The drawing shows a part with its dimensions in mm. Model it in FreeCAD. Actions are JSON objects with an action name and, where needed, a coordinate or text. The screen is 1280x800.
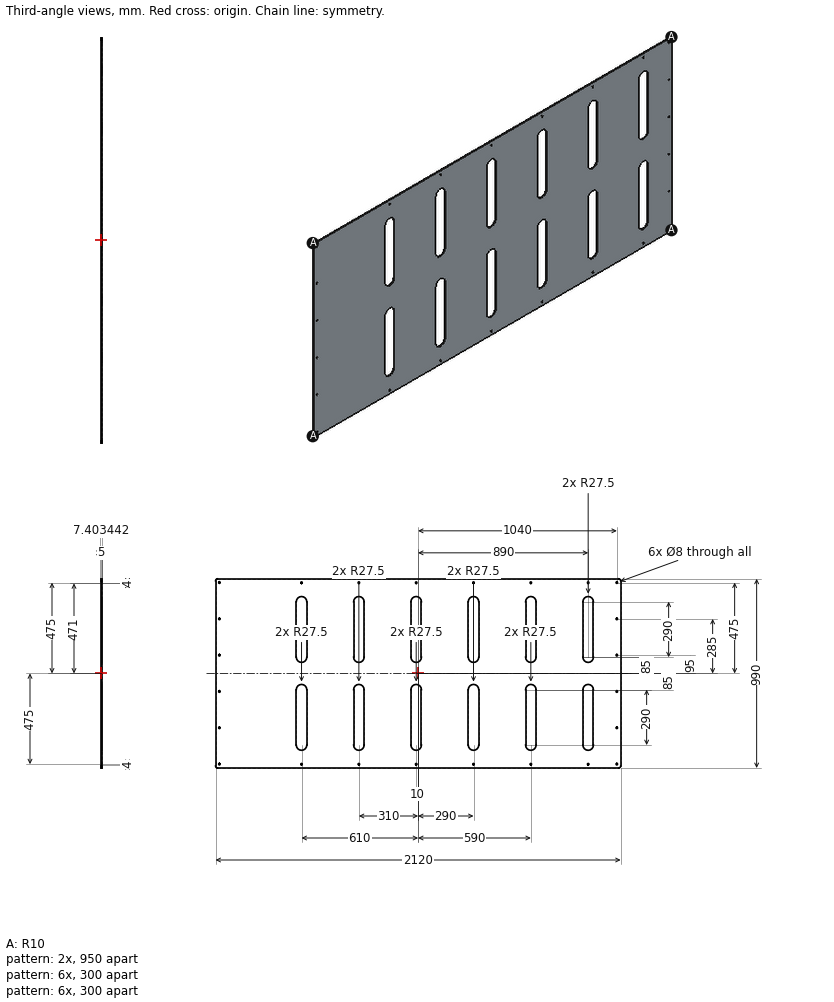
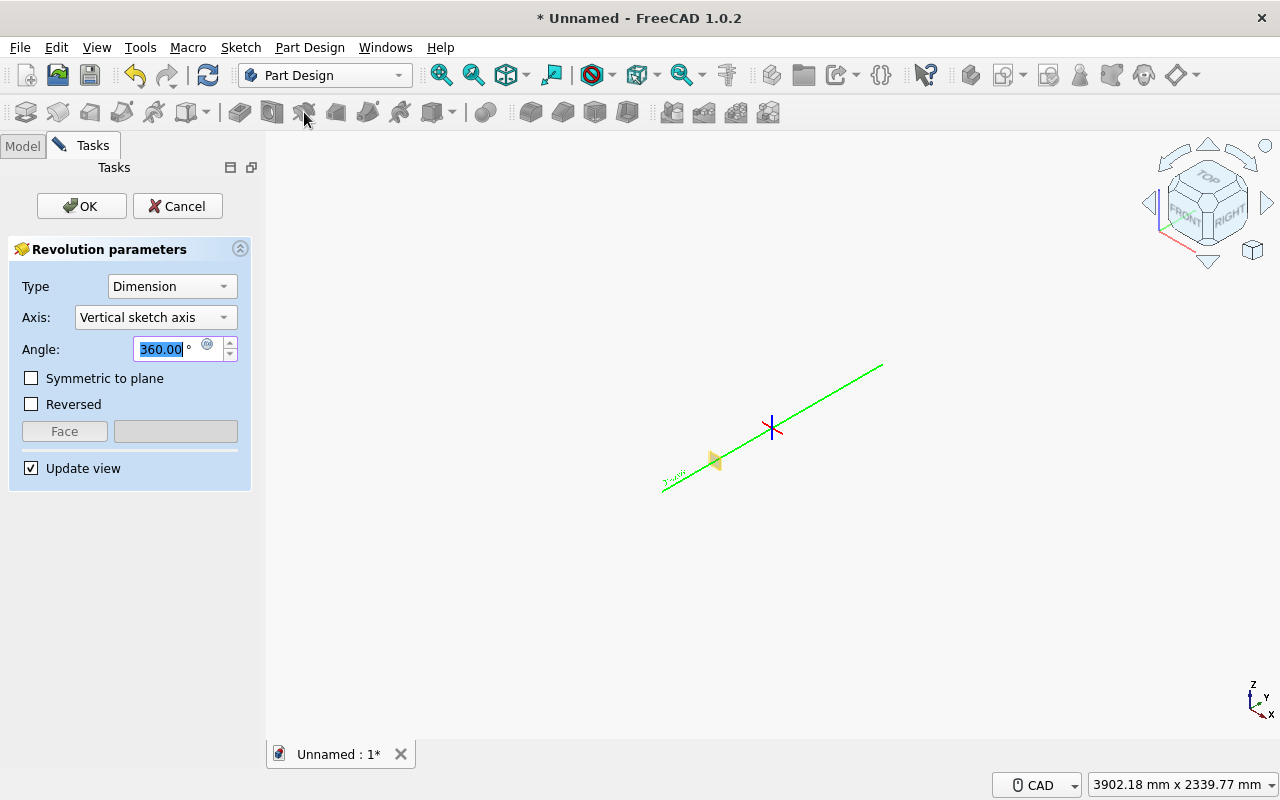
{"action": "left_click", "coordinate": [156, 318]}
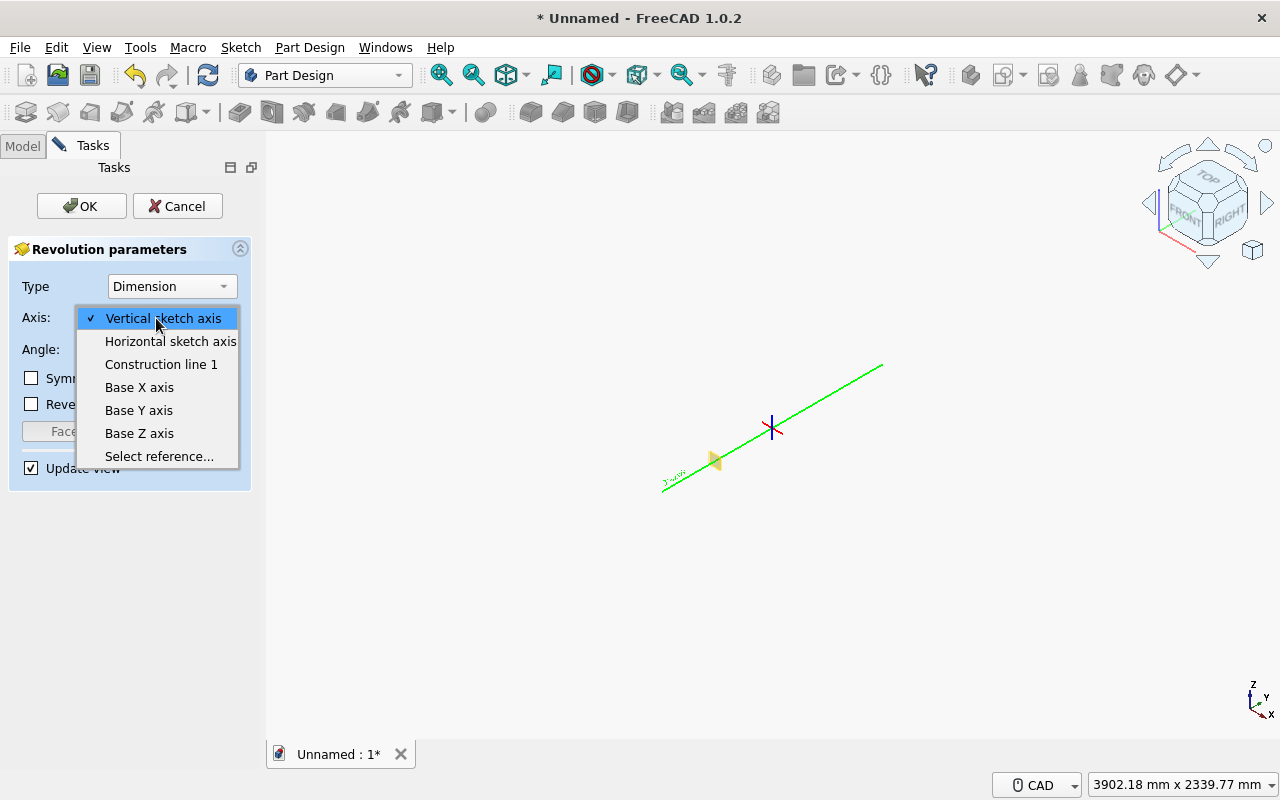
{"action": "left_click", "coordinate": [156, 364]}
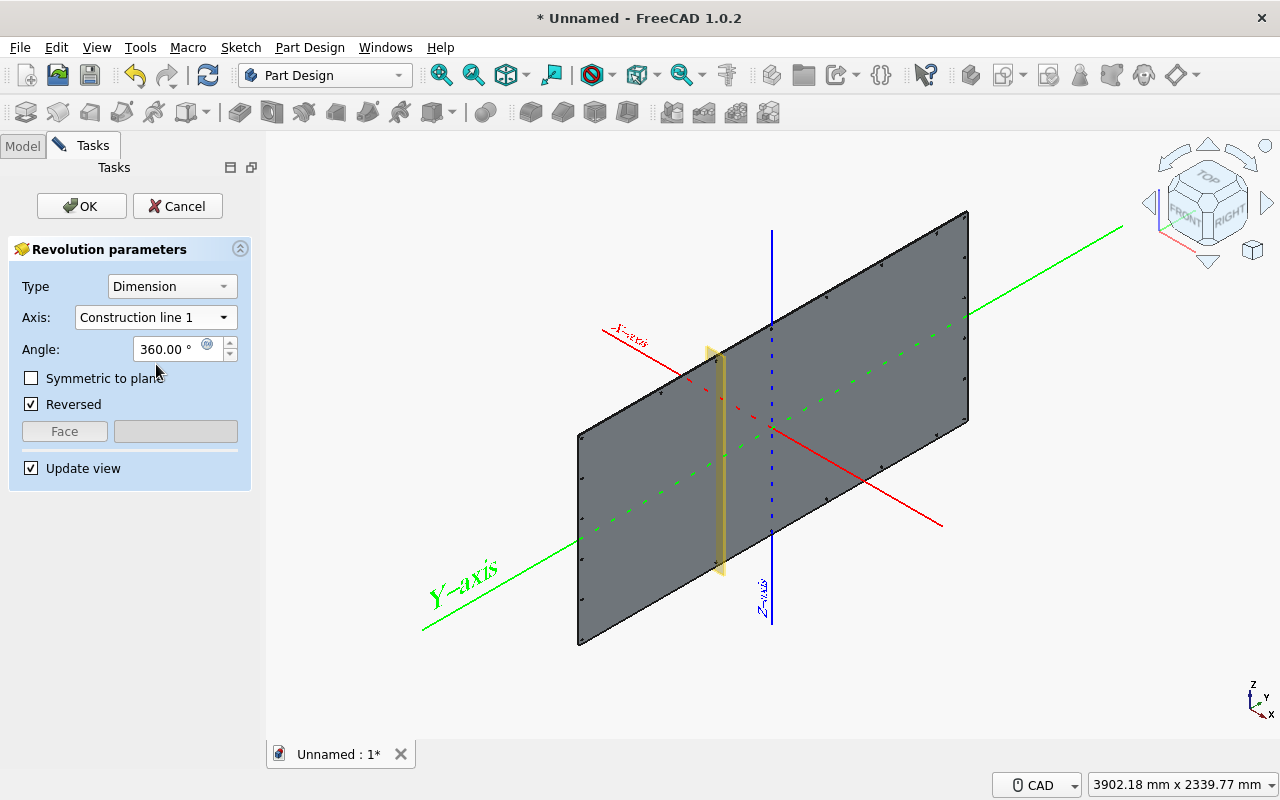
{"action": "left_click", "coordinate": [82, 206]}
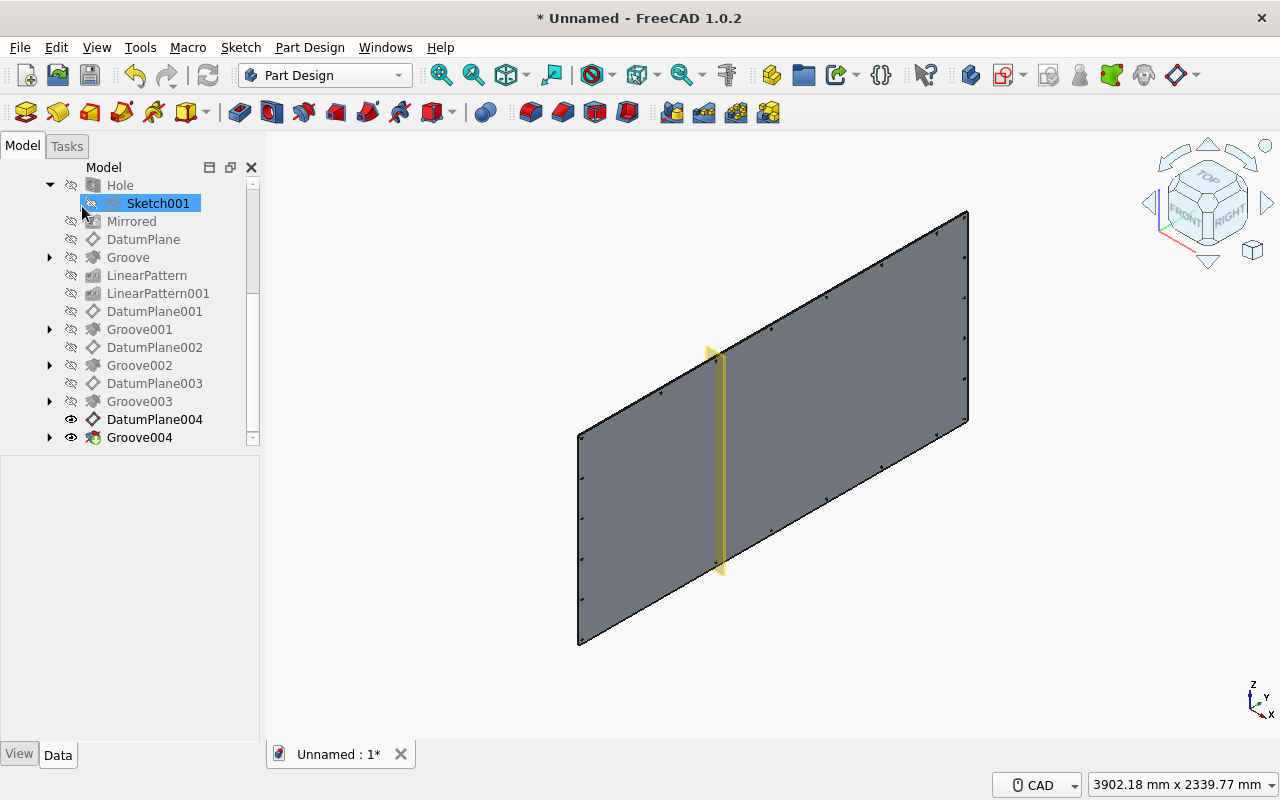
{"action": "left_click", "coordinate": [116, 419]}
{"action": "key", "text": "space"}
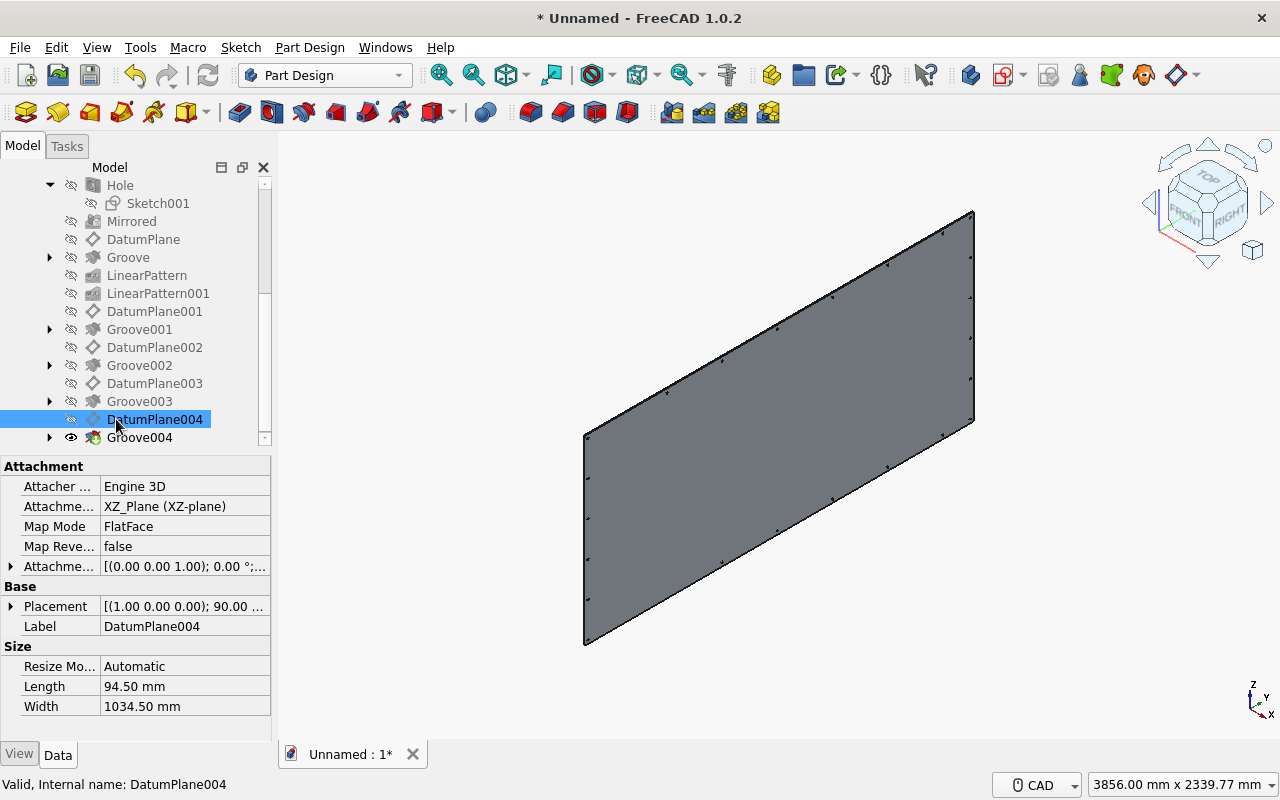
{"action": "scroll", "coordinate": [140, 307], "scroll_direction": "down", "scroll_amount": 3}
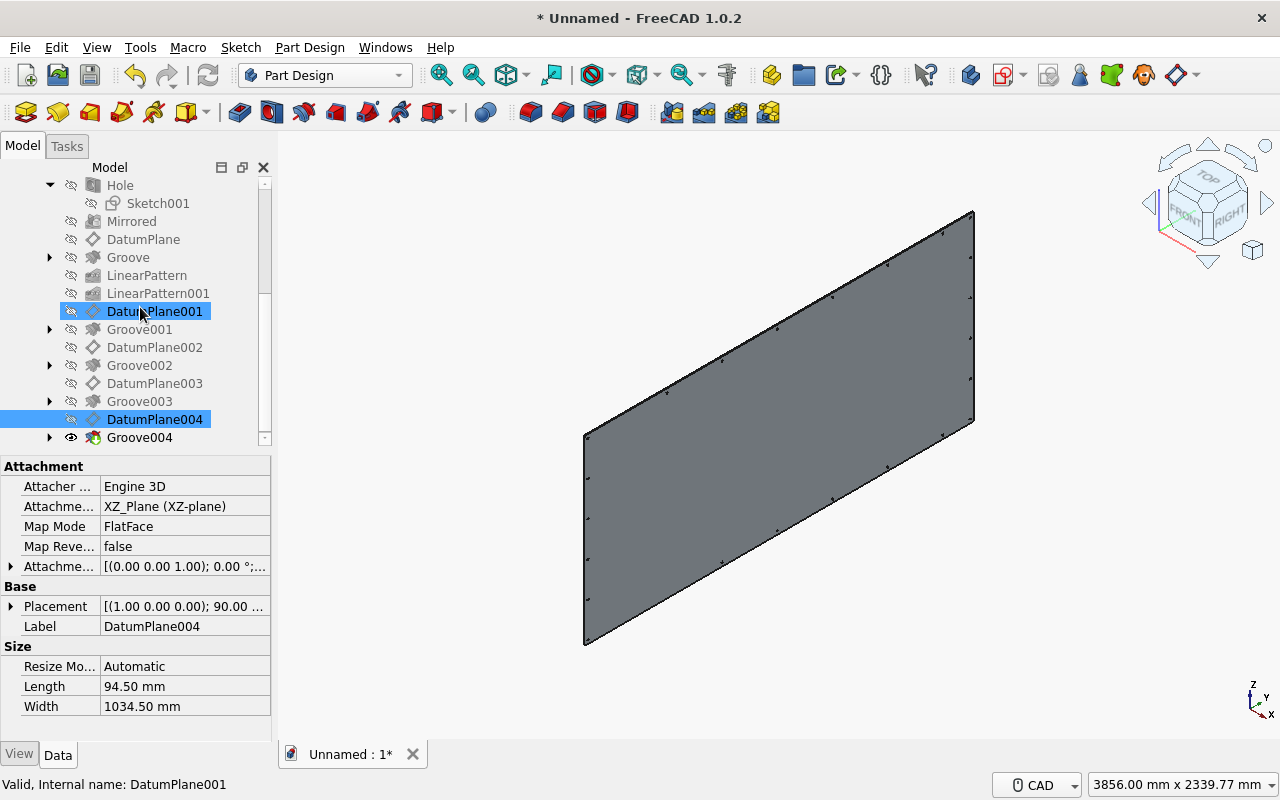
{"action": "scroll", "coordinate": [140, 307], "scroll_direction": "up", "scroll_amount": 15}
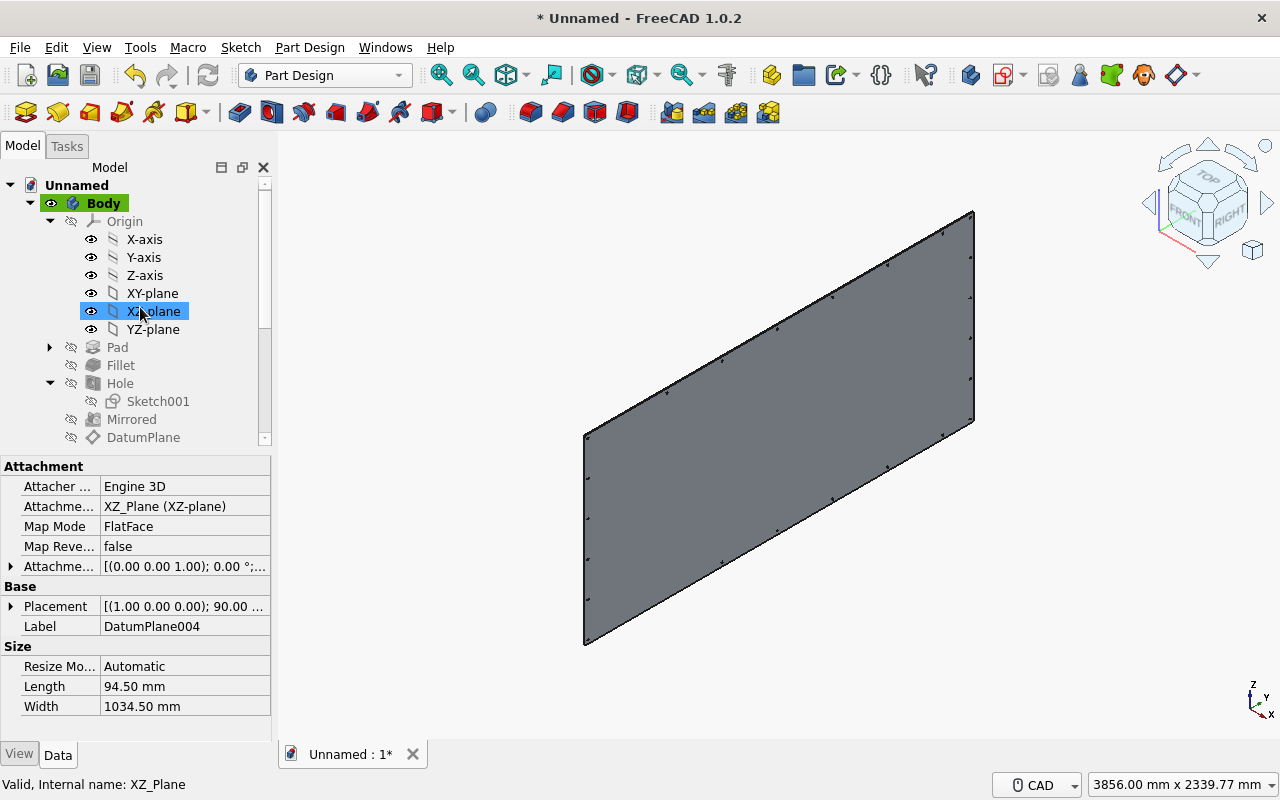
{"action": "left_click", "coordinate": [136, 311]}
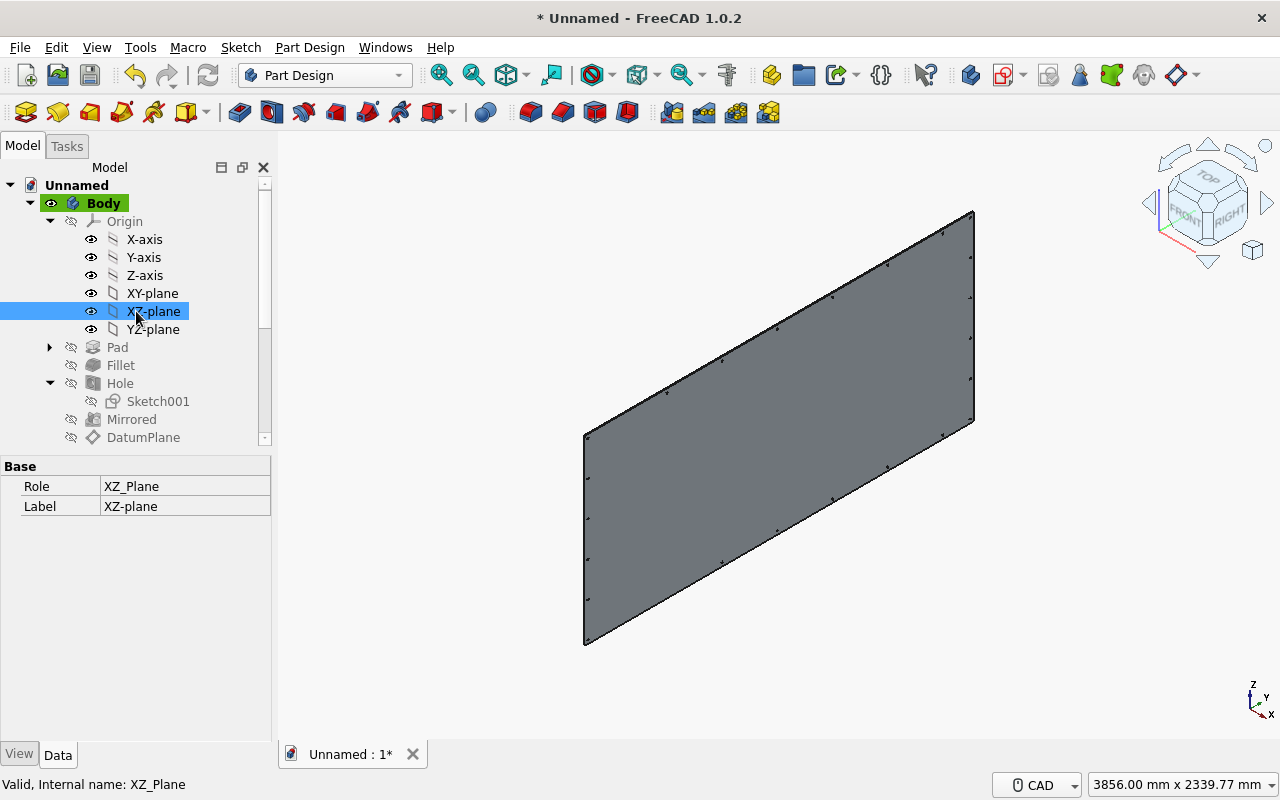
{"action": "left_click", "coordinate": [1176, 76]}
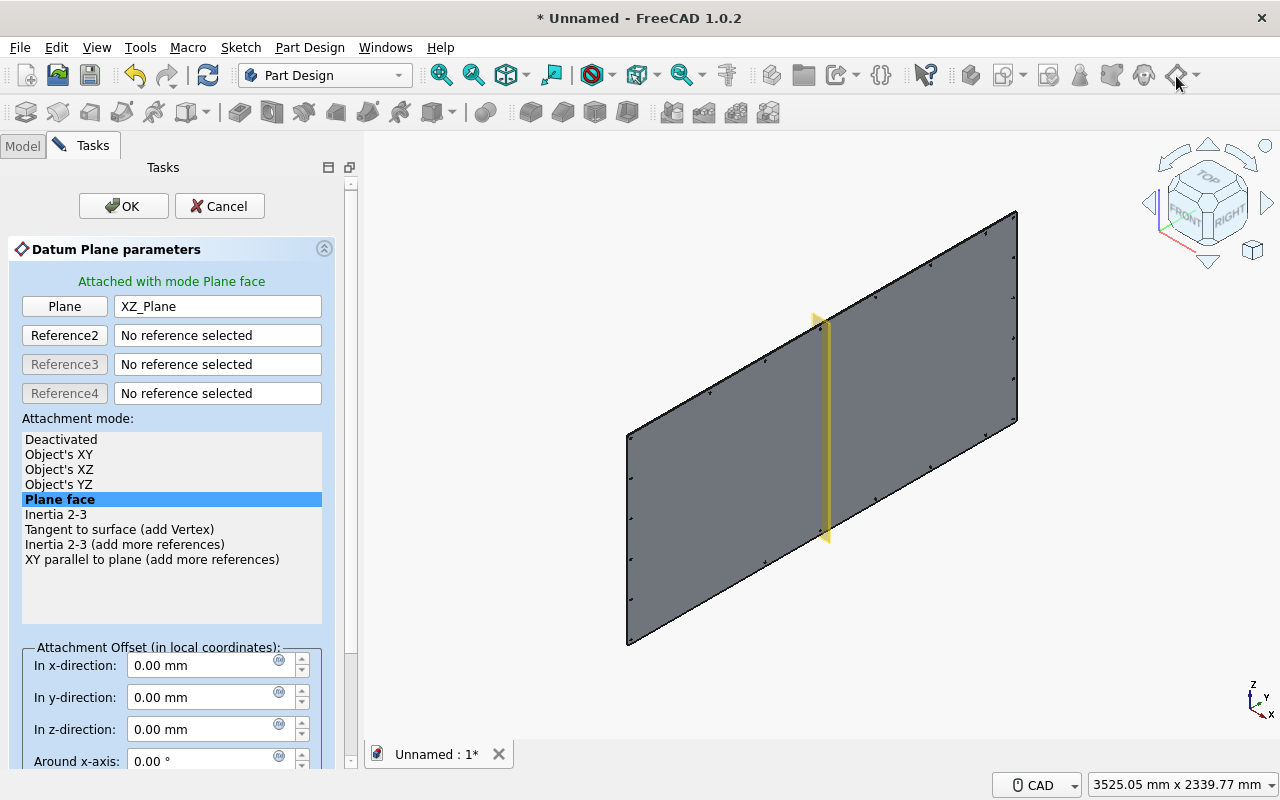
{"action": "triple_click", "coordinate": [210, 729]}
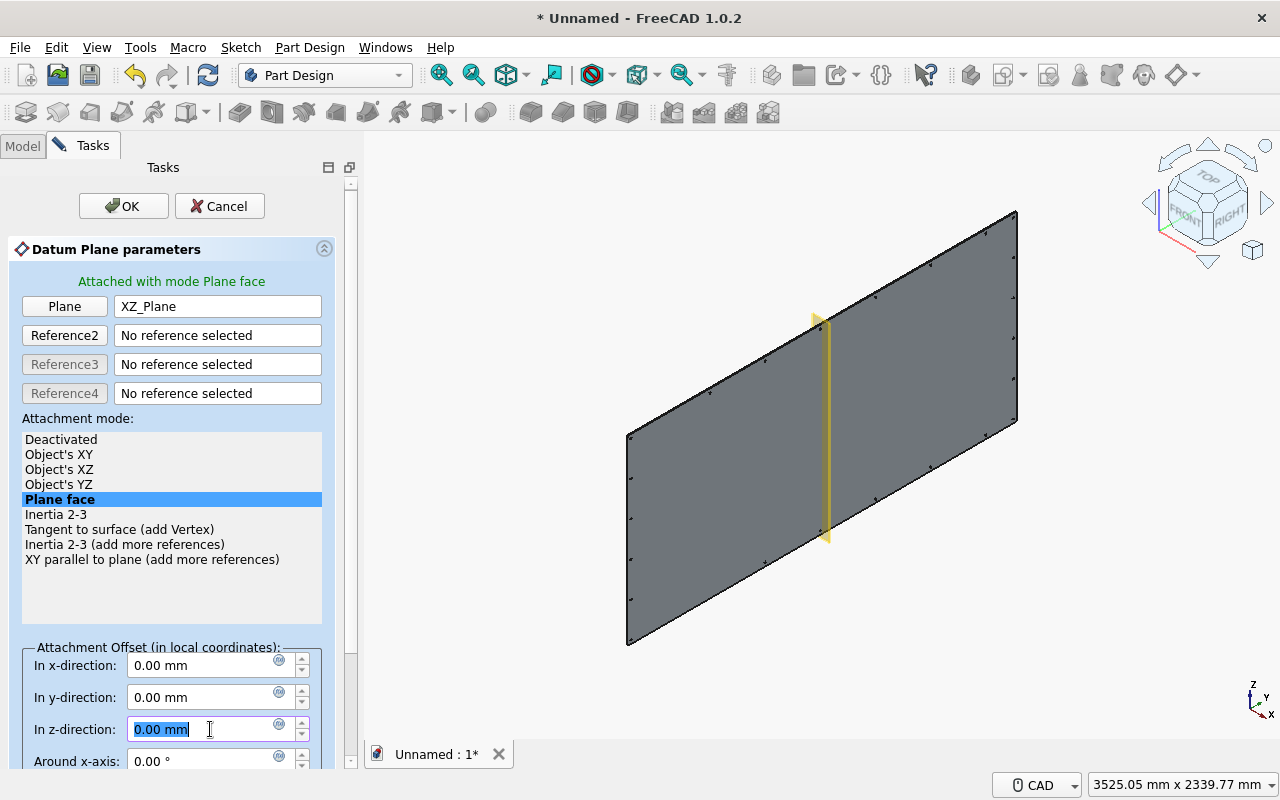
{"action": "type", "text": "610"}
{"action": "key", "text": "Tab"}